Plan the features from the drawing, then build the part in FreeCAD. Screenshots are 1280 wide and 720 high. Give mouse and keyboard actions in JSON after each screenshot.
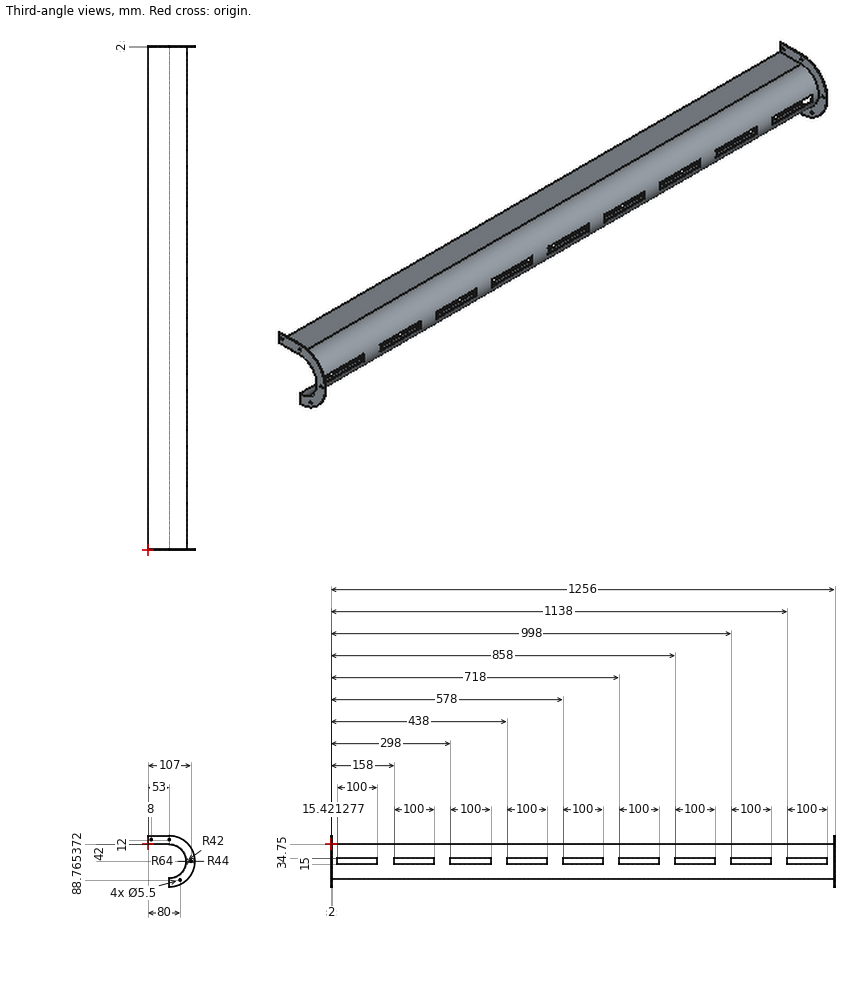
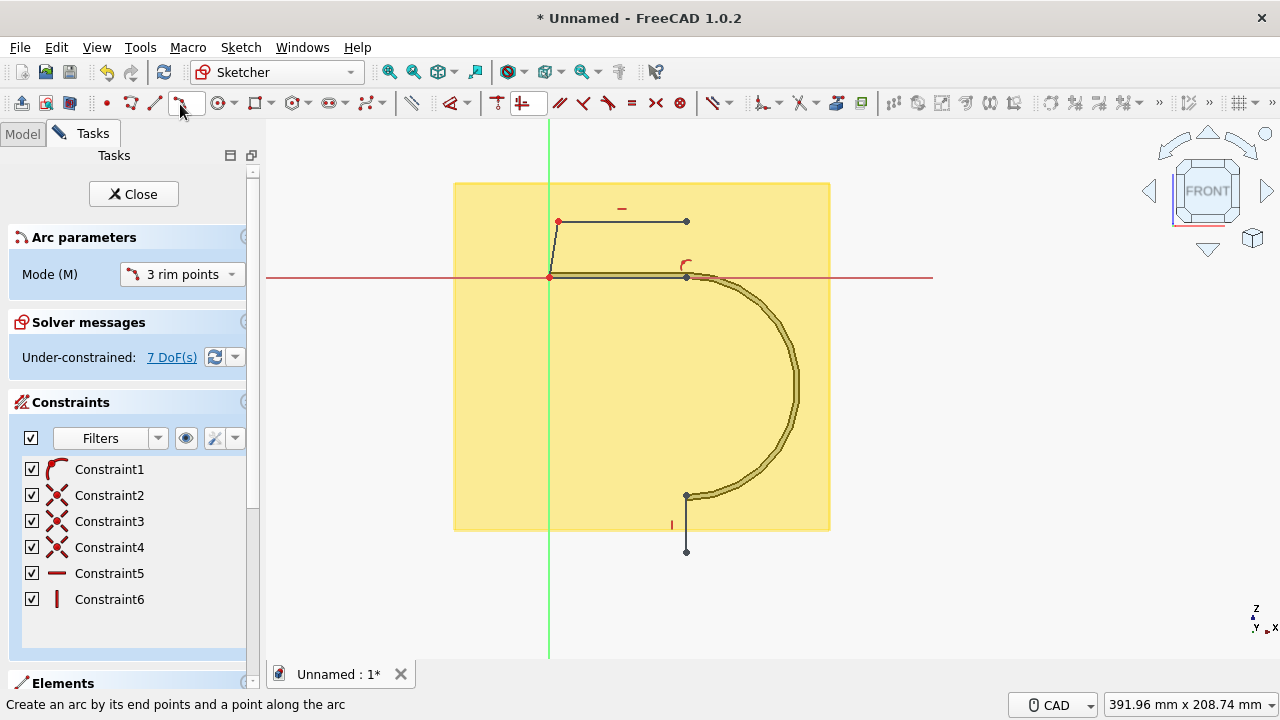
{"action": "left_click", "coordinate": [686, 222]}
{"action": "left_click", "coordinate": [686, 553]}
{"action": "left_click", "coordinate": [852, 386]}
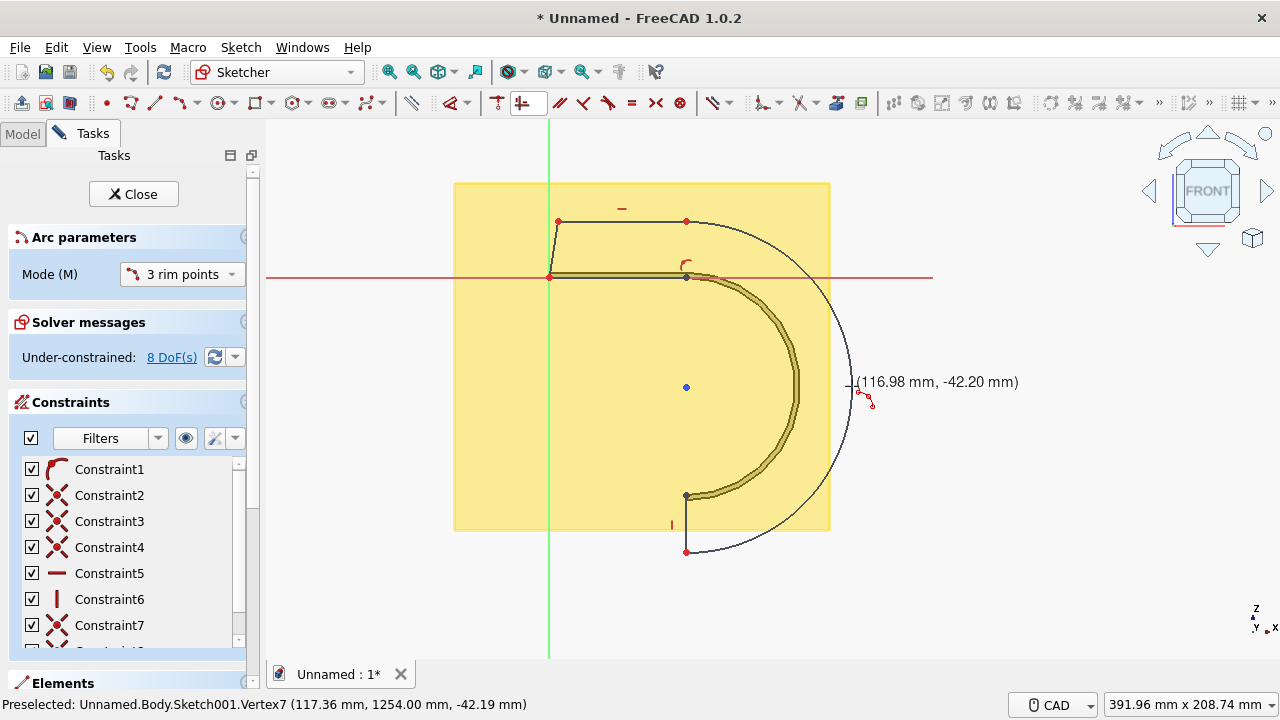
{"action": "left_click", "coordinate": [686, 496]}
{"action": "left_click", "coordinate": [686, 278]}
{"action": "left_click", "coordinate": [795, 386]}
{"action": "key", "text": "Escape"}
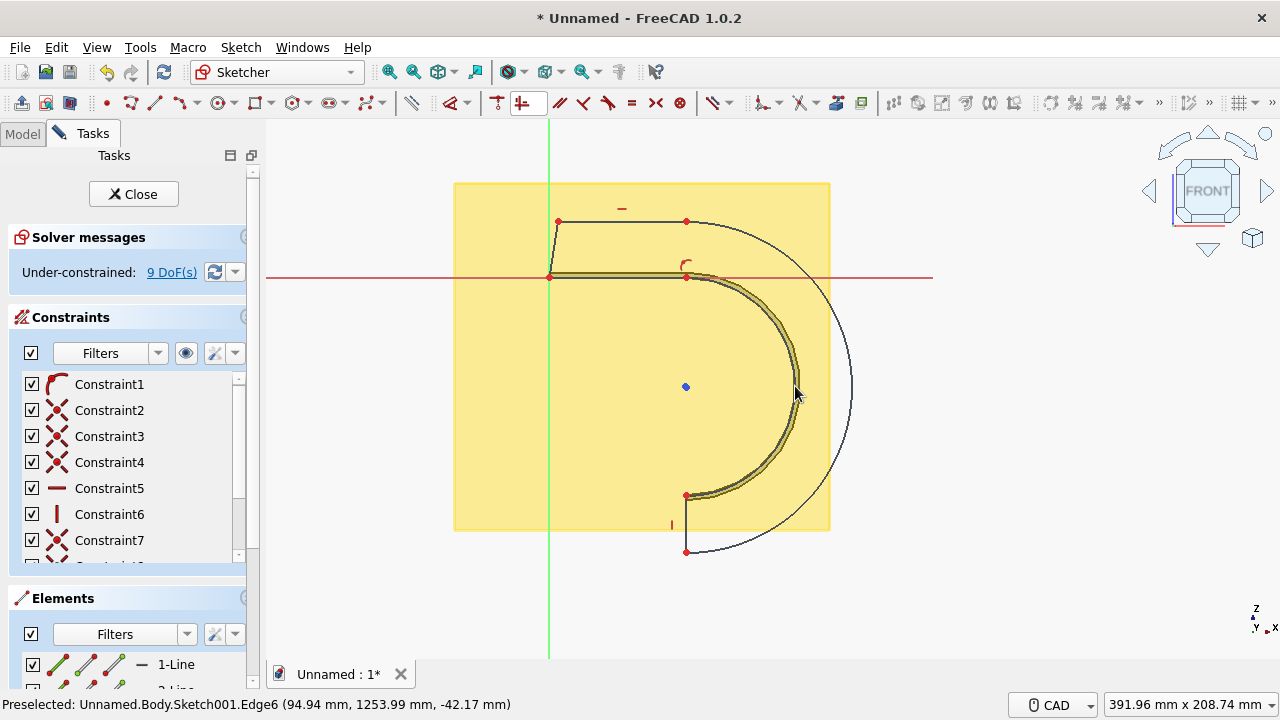
{"action": "left_click", "coordinate": [552, 261]}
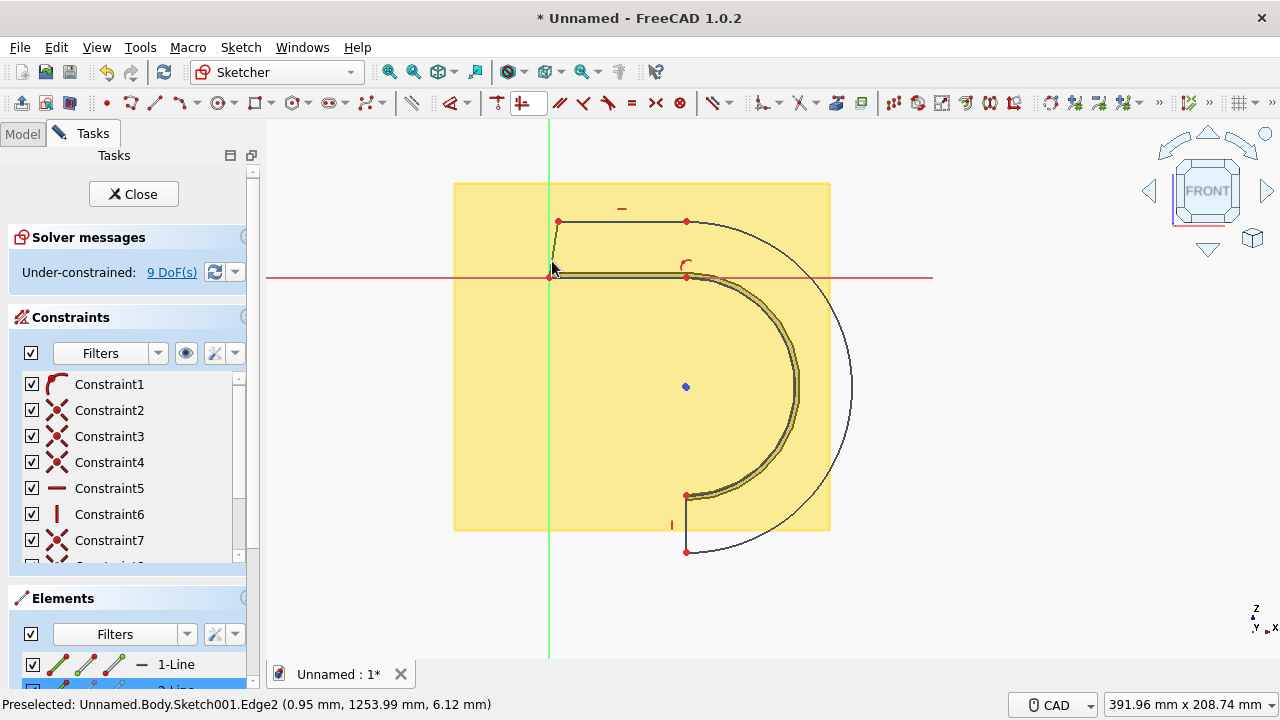
{"action": "key", "text": "v"}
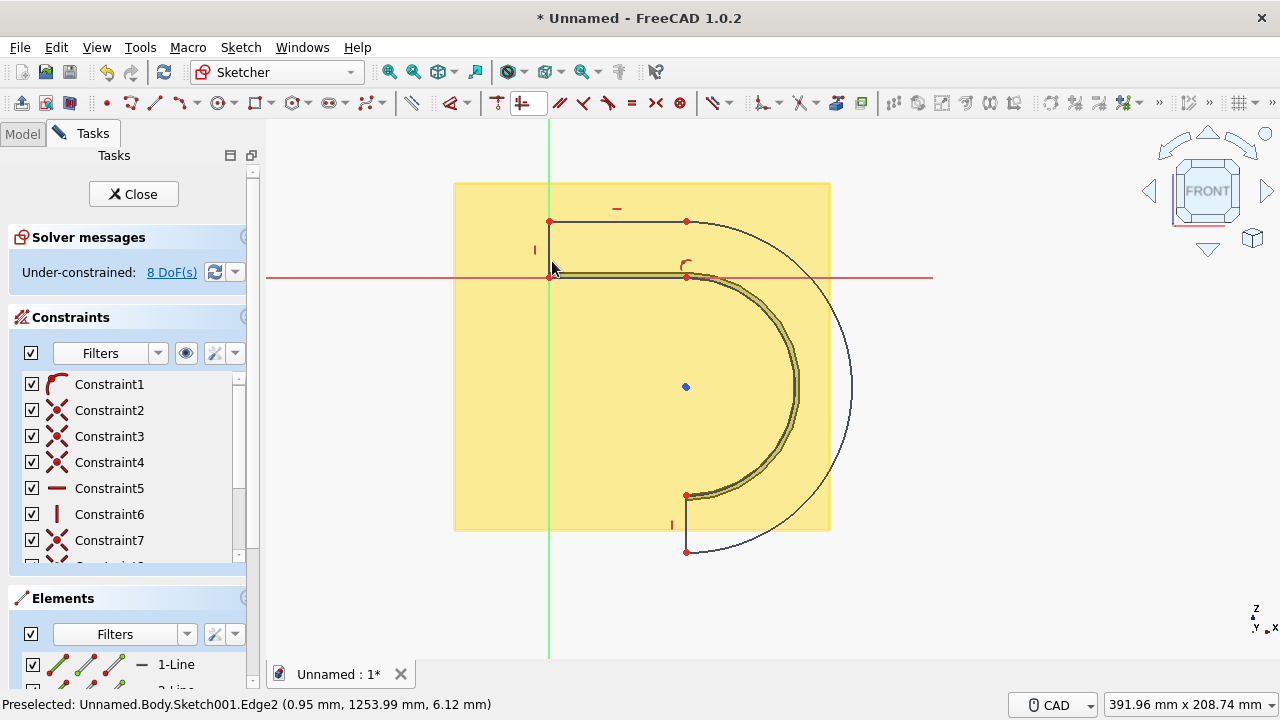
{"action": "left_click", "coordinate": [820, 485]}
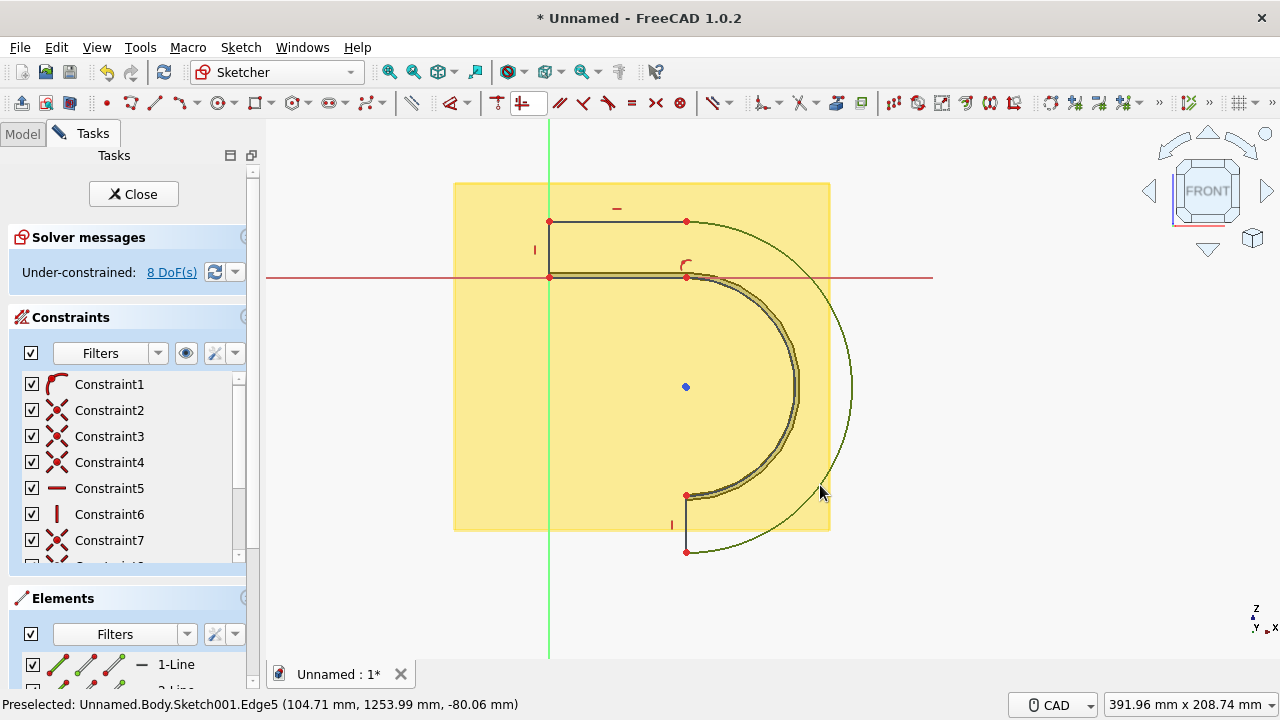
{"action": "left_click", "coordinate": [774, 451]}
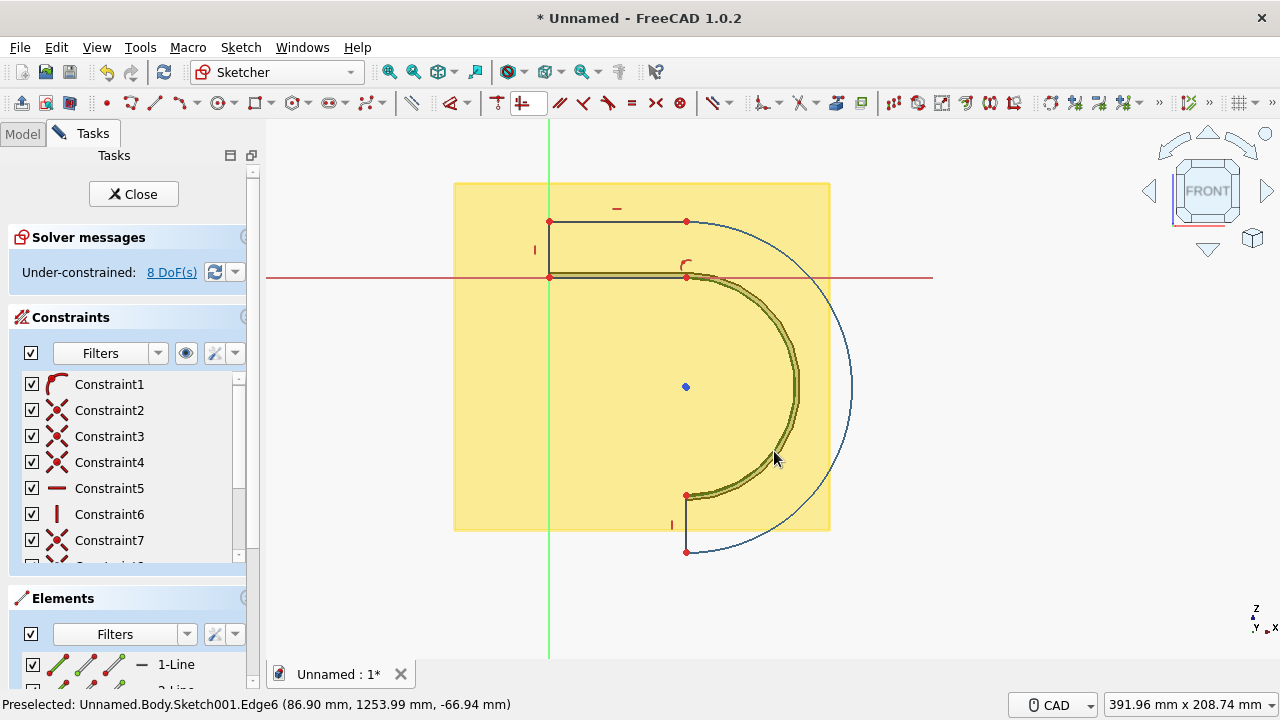
{"action": "left_click", "coordinate": [498, 104]}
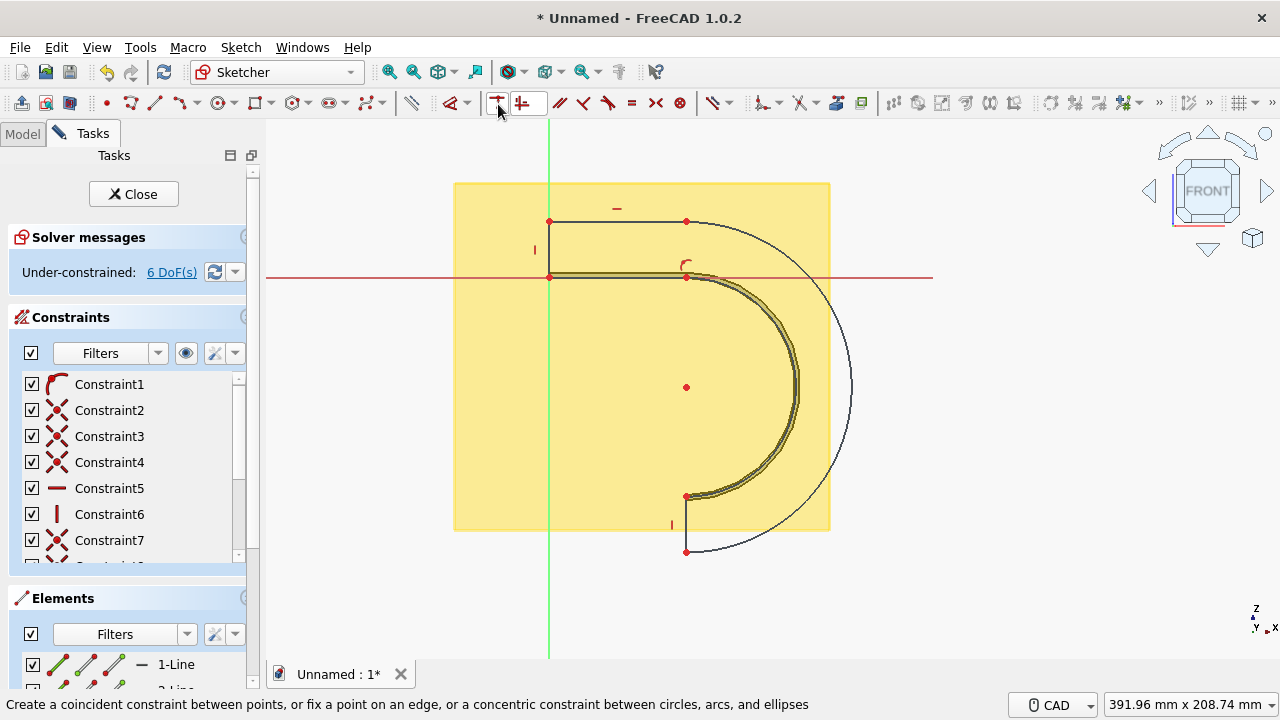
{"action": "left_click", "coordinate": [450, 104]}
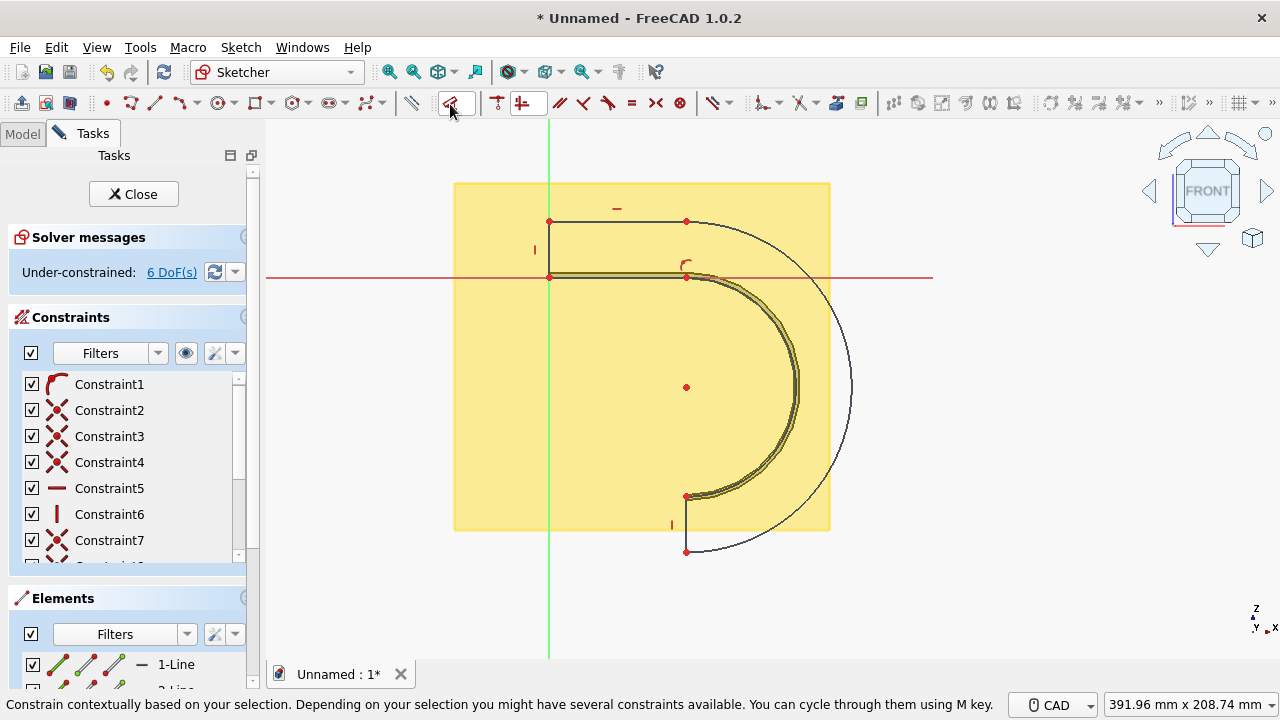
{"action": "left_click", "coordinate": [820, 485]}
{"action": "left_click", "coordinate": [846, 504]}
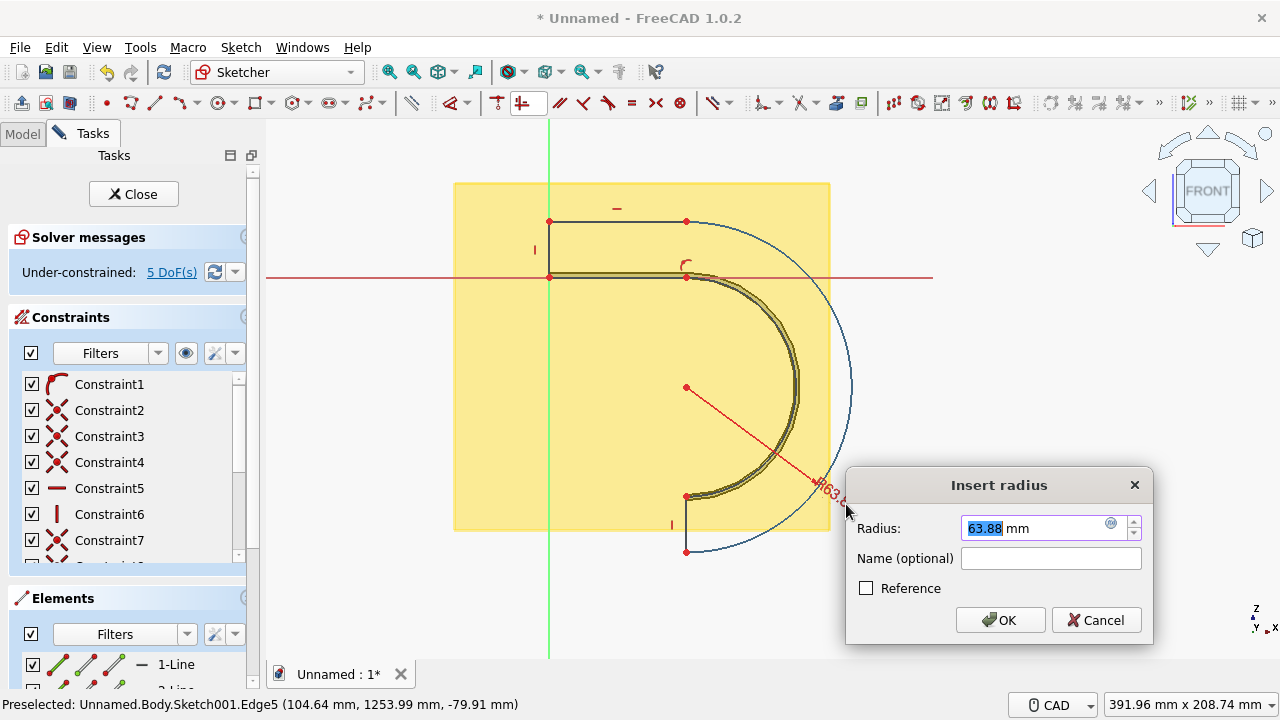
{"action": "type", "text": "64"}
{"action": "key", "text": "Return"}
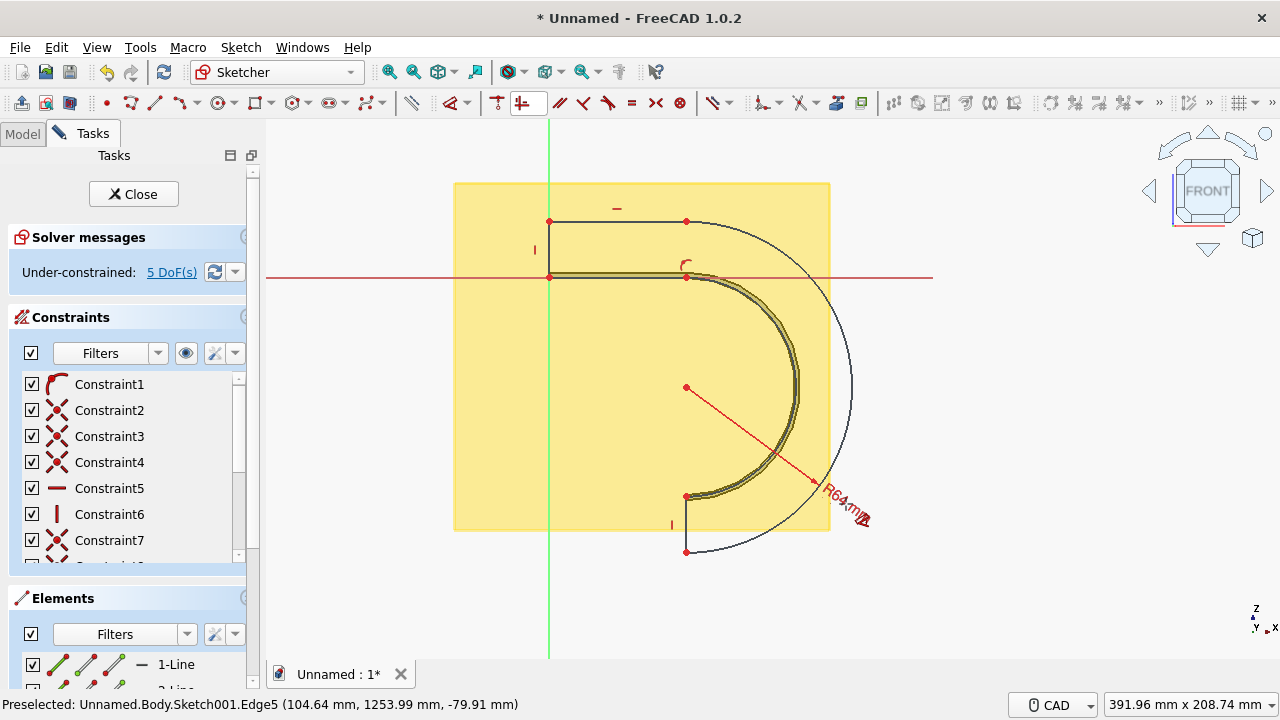
{"action": "left_click", "coordinate": [775, 452]}
{"action": "left_click", "coordinate": [801, 471]}